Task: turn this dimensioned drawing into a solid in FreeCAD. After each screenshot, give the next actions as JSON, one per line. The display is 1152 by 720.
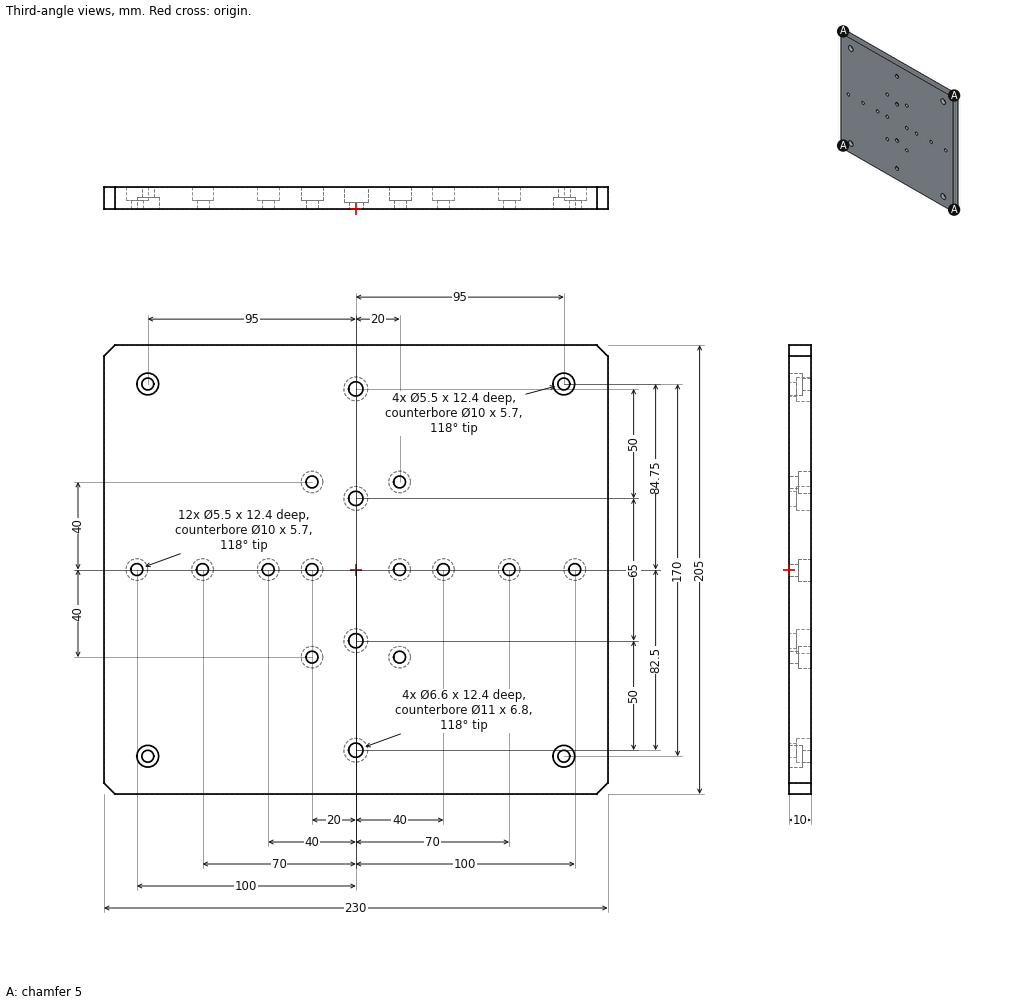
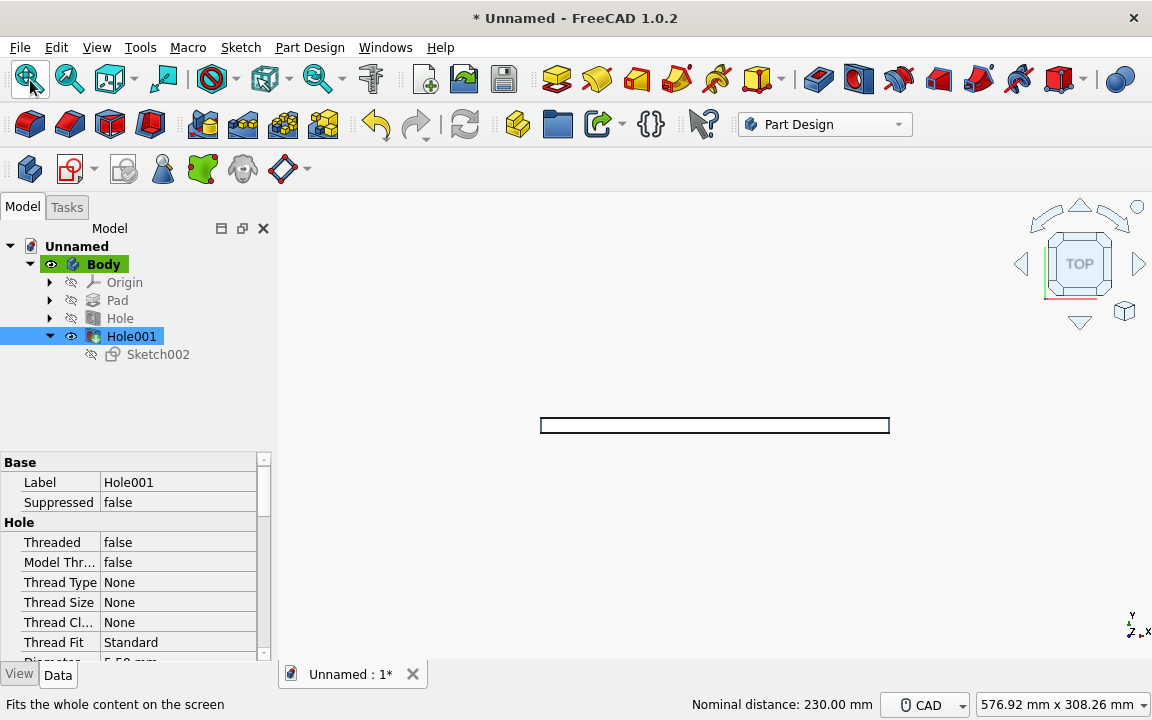
{"action": "key", "text": "1"}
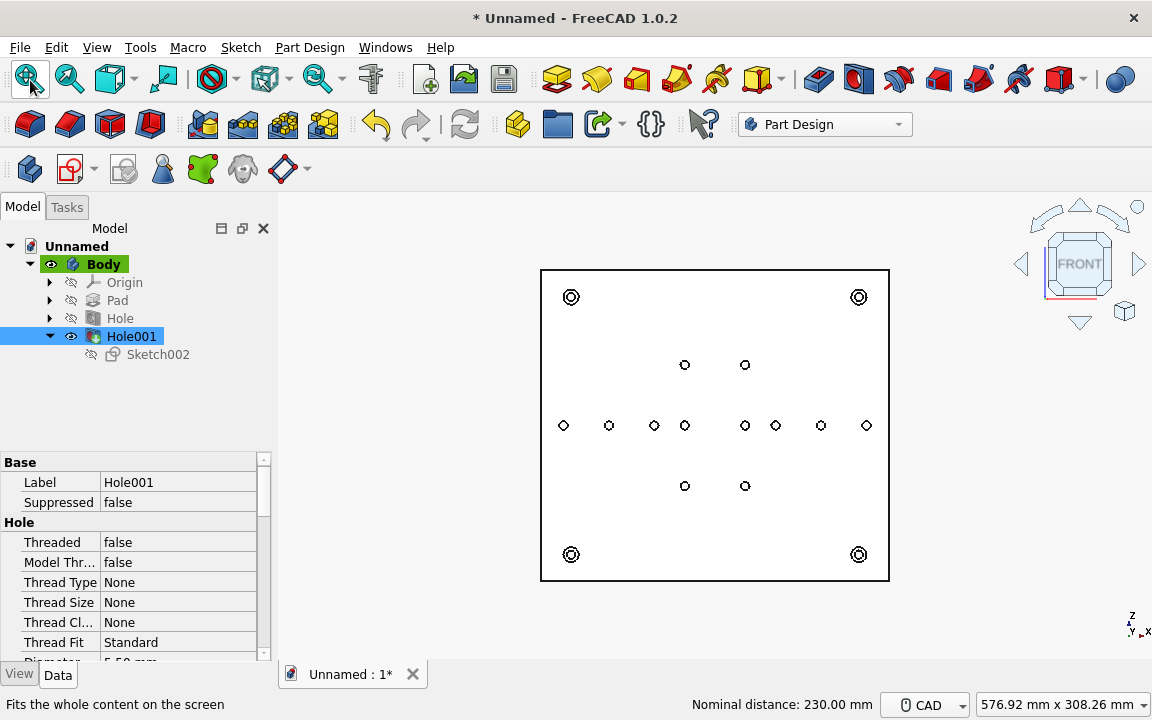
{"action": "scroll", "coordinate": [541, 580], "scroll_direction": "up", "scroll_amount": 5}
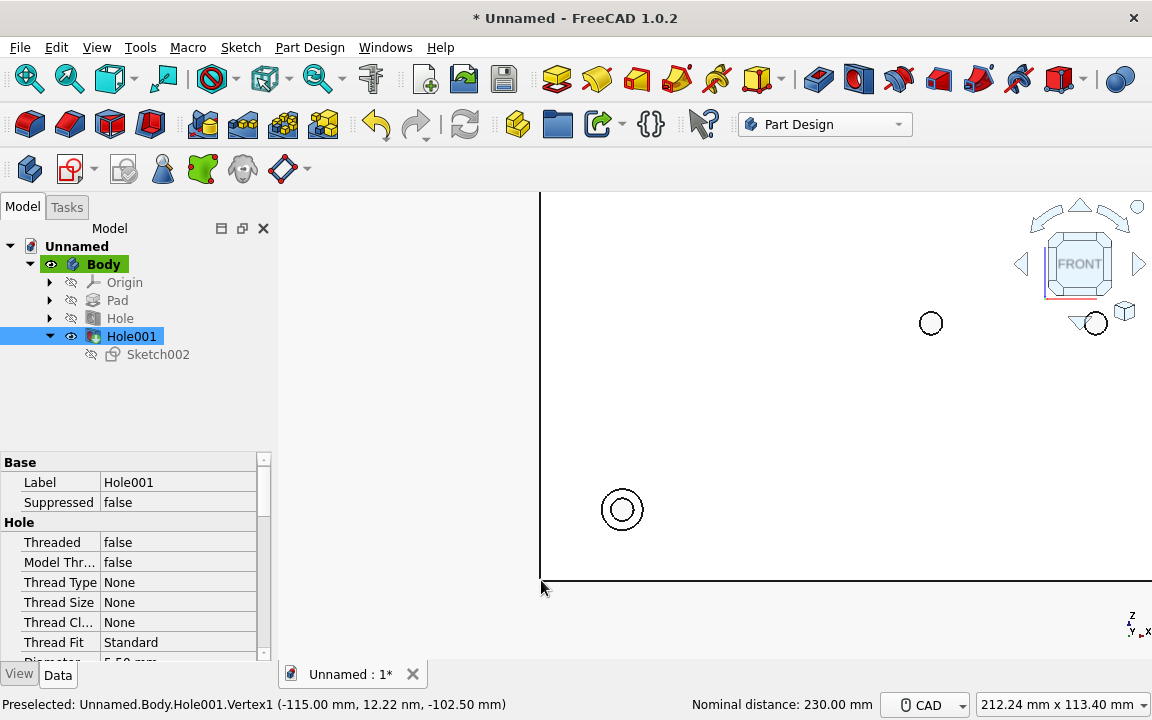
{"action": "left_click", "coordinate": [30, 80]}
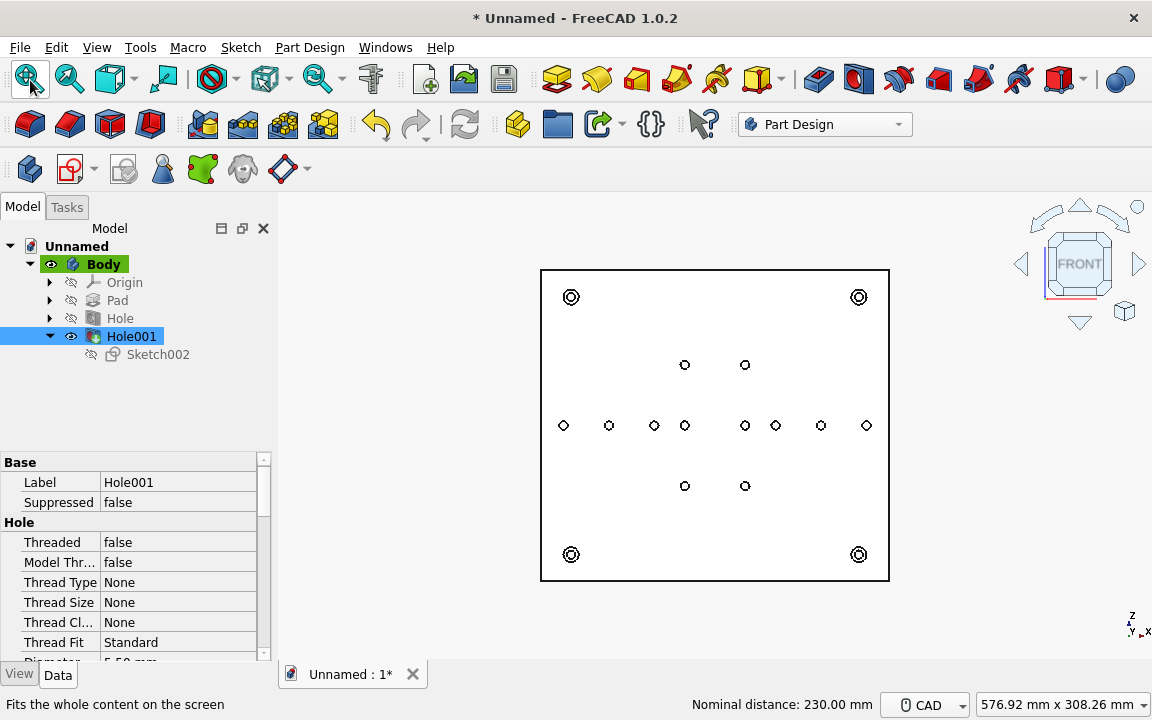
{"action": "key", "text": "3"}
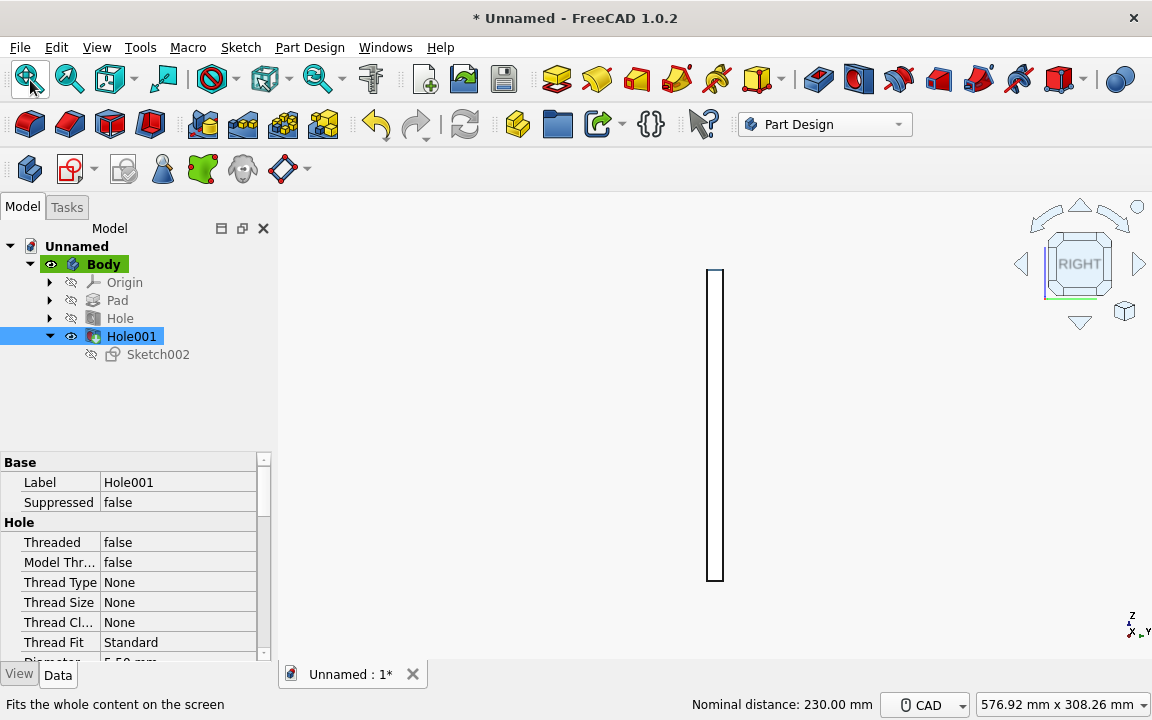
{"action": "left_click", "coordinate": [715, 580], "text": "ctrl"}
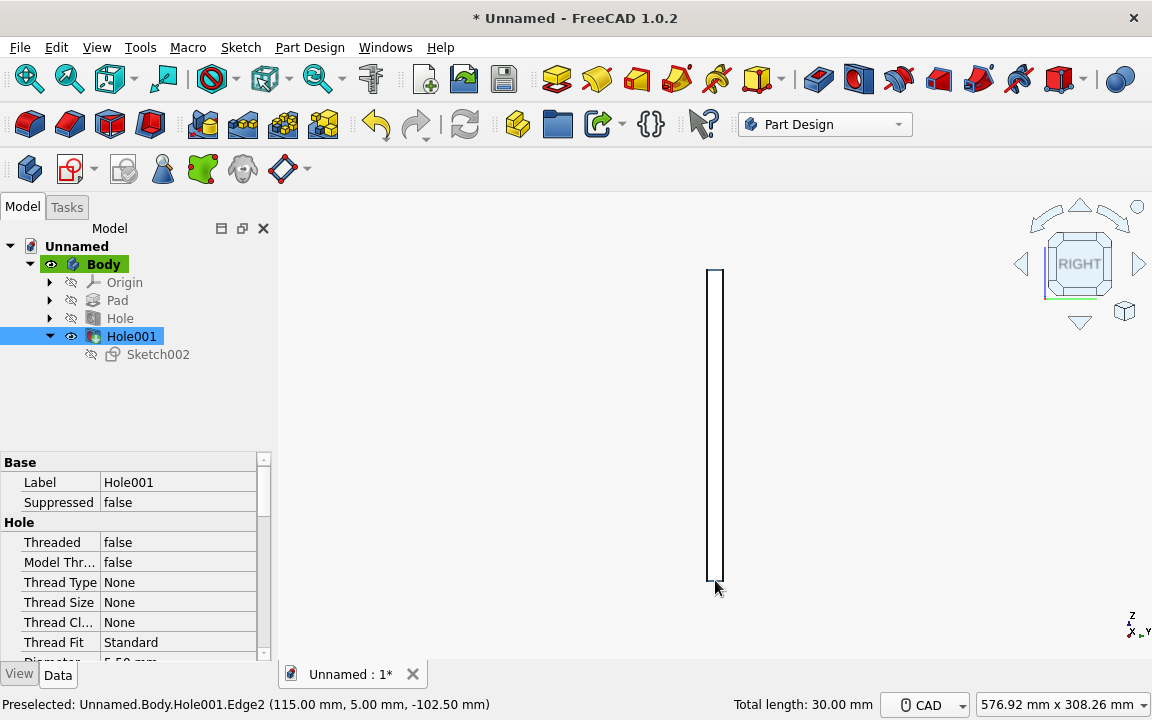
{"action": "scroll", "coordinate": [715, 580], "scroll_direction": "up", "scroll_amount": 5}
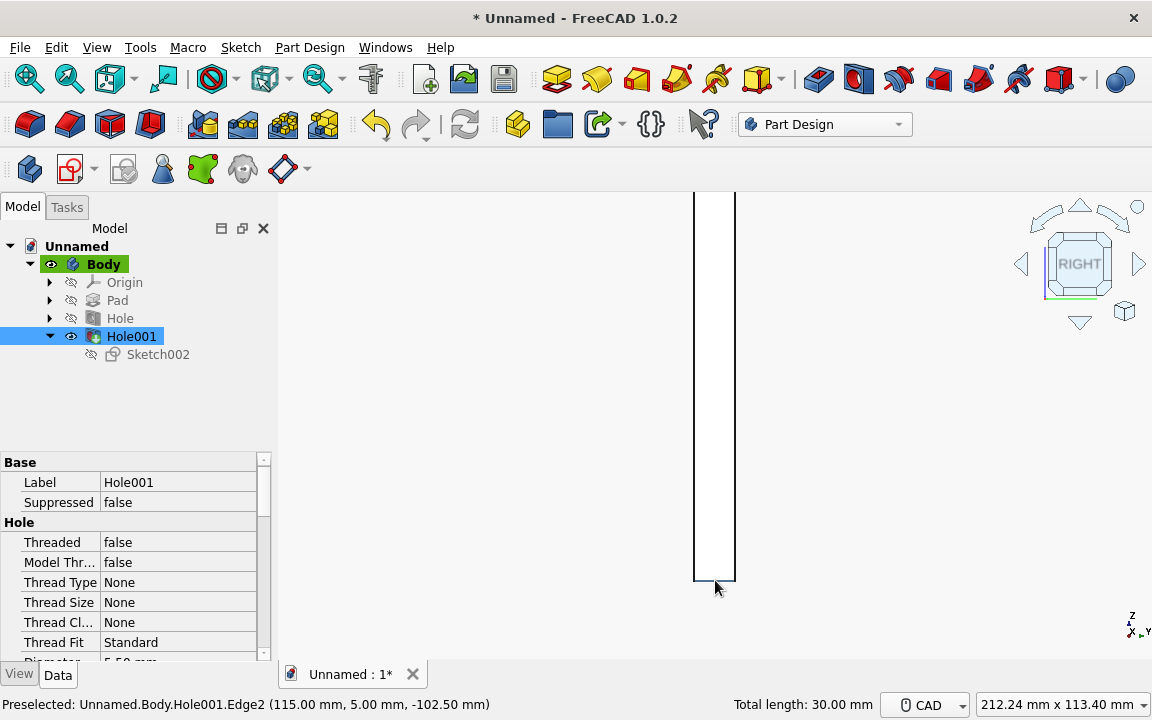
{"action": "left_click", "coordinate": [30, 80]}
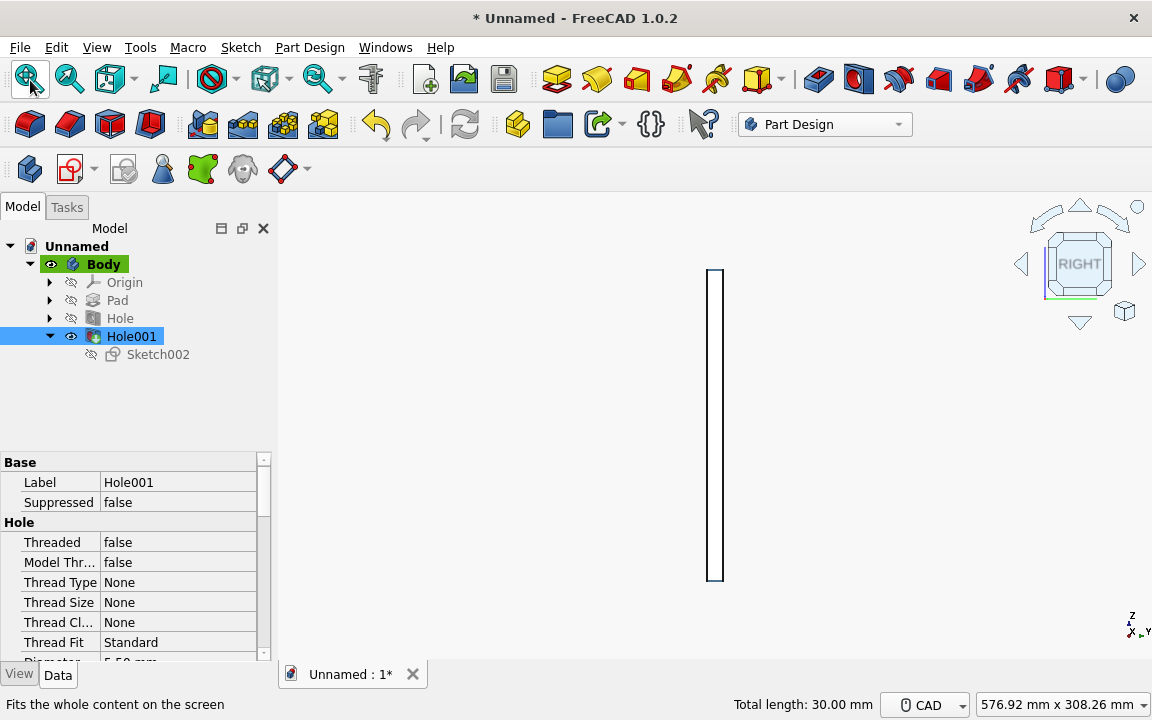
{"action": "key", "text": "5"}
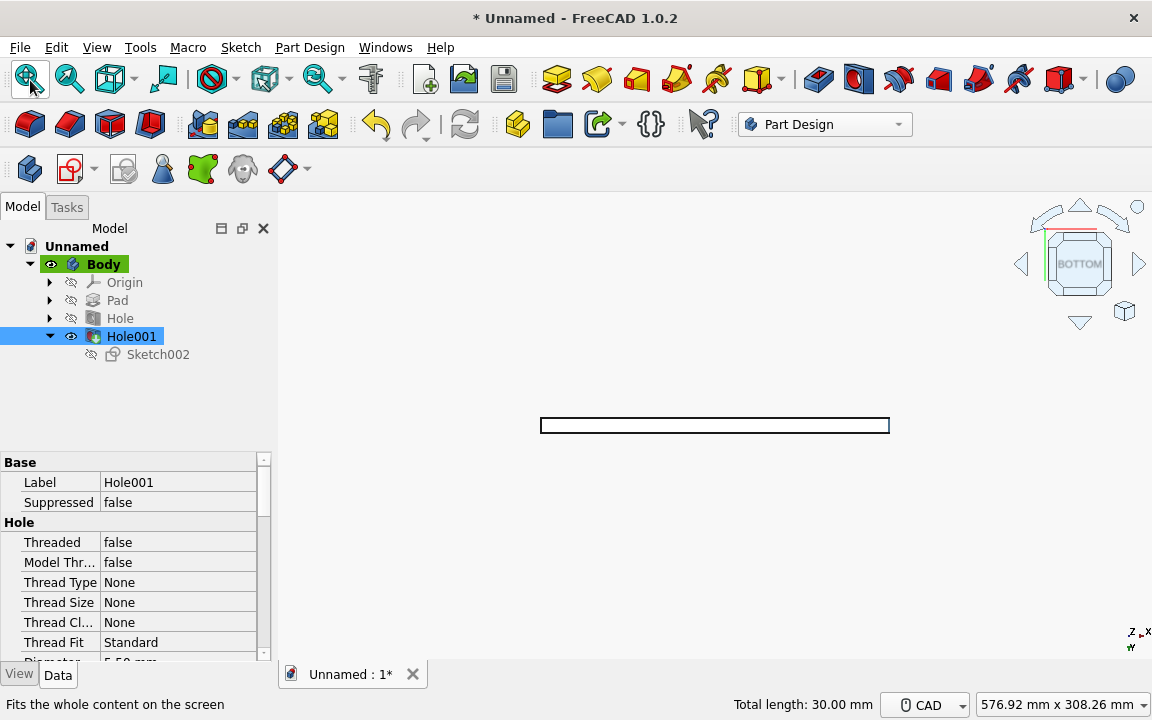
{"action": "left_click", "coordinate": [30, 80]}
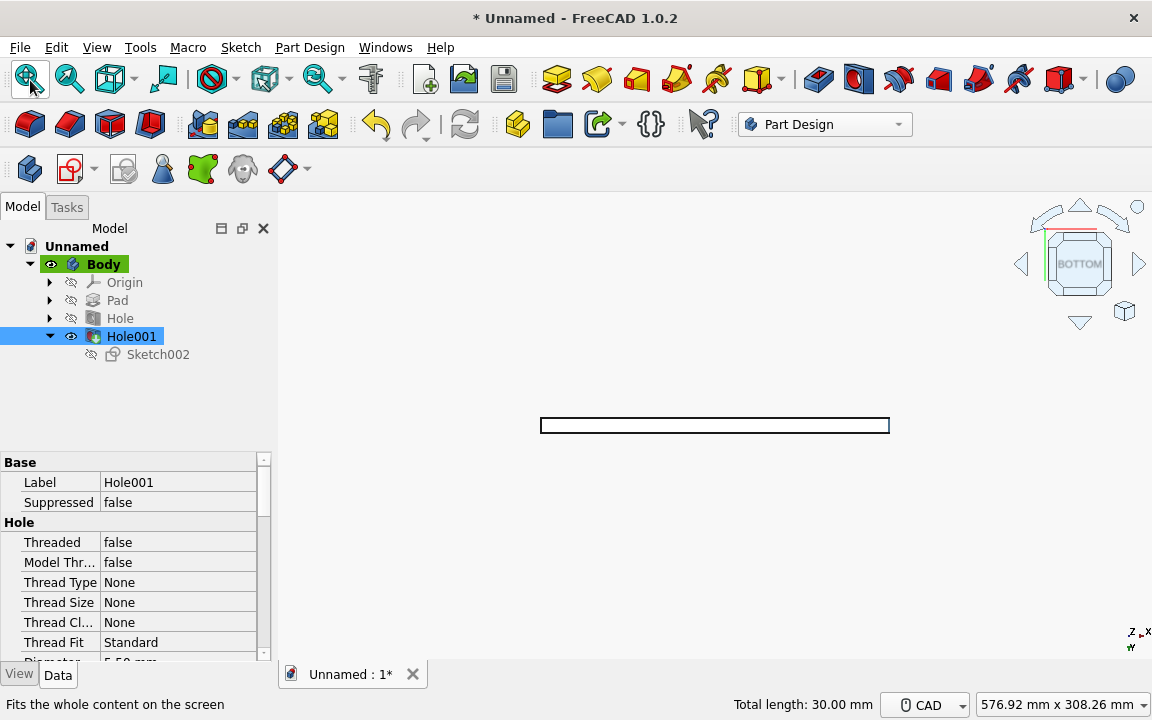
{"action": "left_click", "coordinate": [541, 424], "text": "ctrl"}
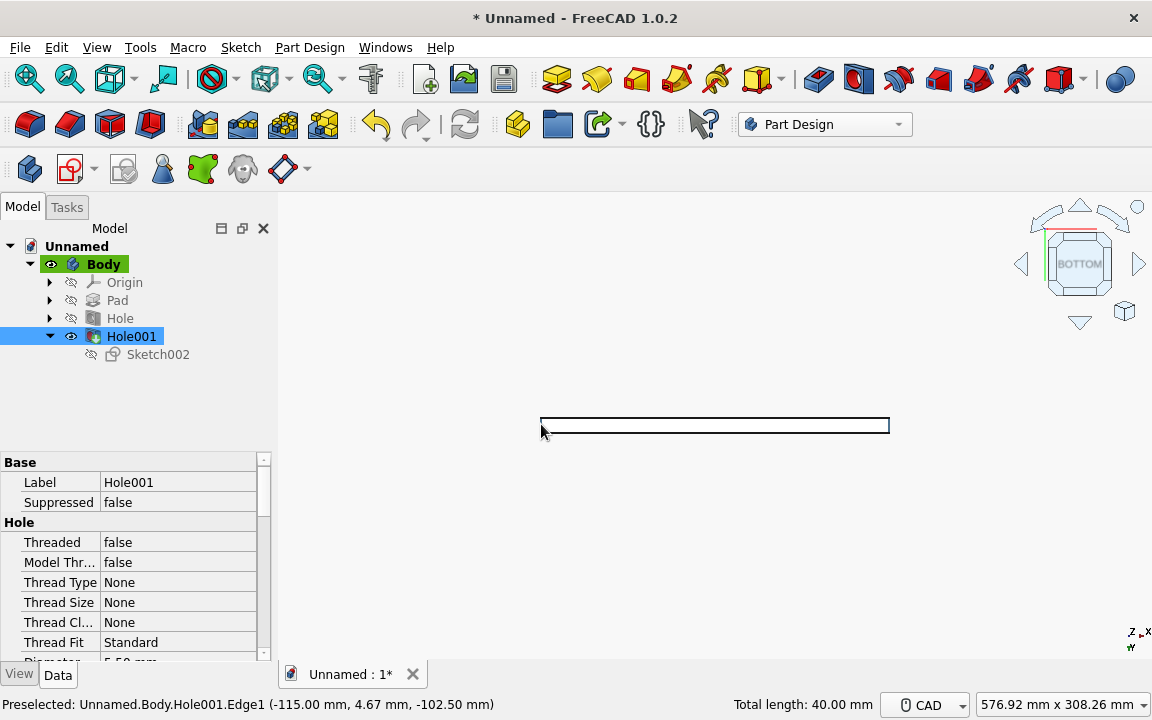
{"action": "left_click", "coordinate": [70, 124]}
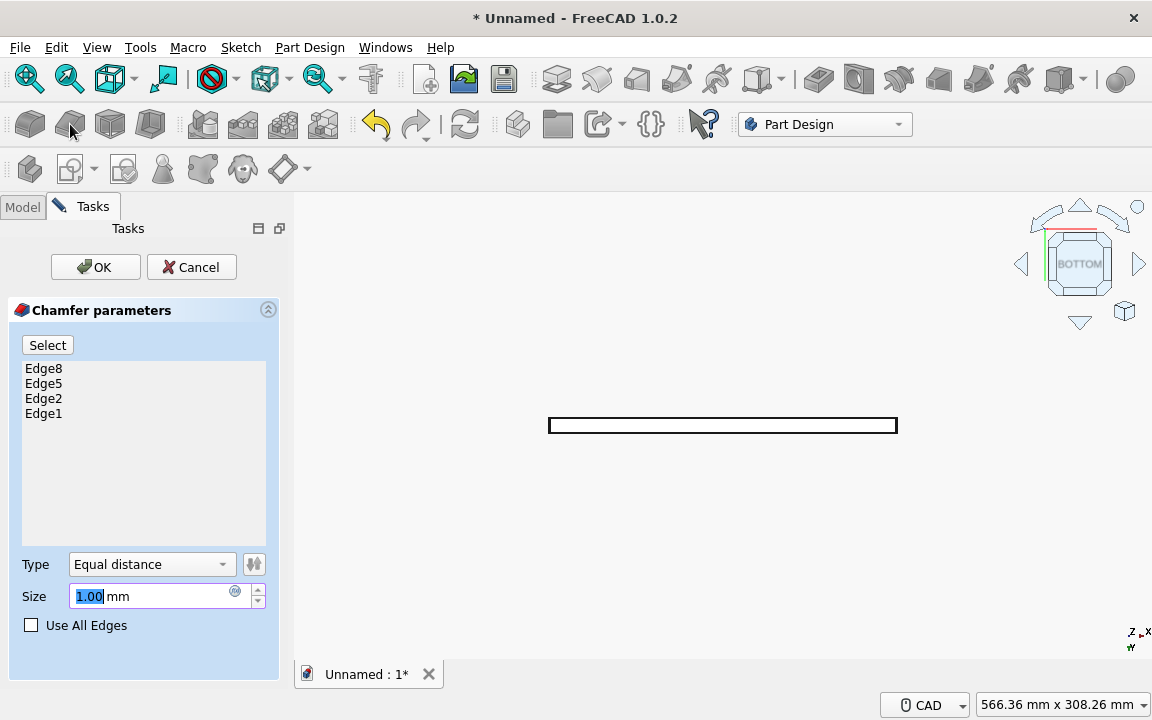
{"action": "type", "text": "5"}
{"action": "key", "text": "Tab"}